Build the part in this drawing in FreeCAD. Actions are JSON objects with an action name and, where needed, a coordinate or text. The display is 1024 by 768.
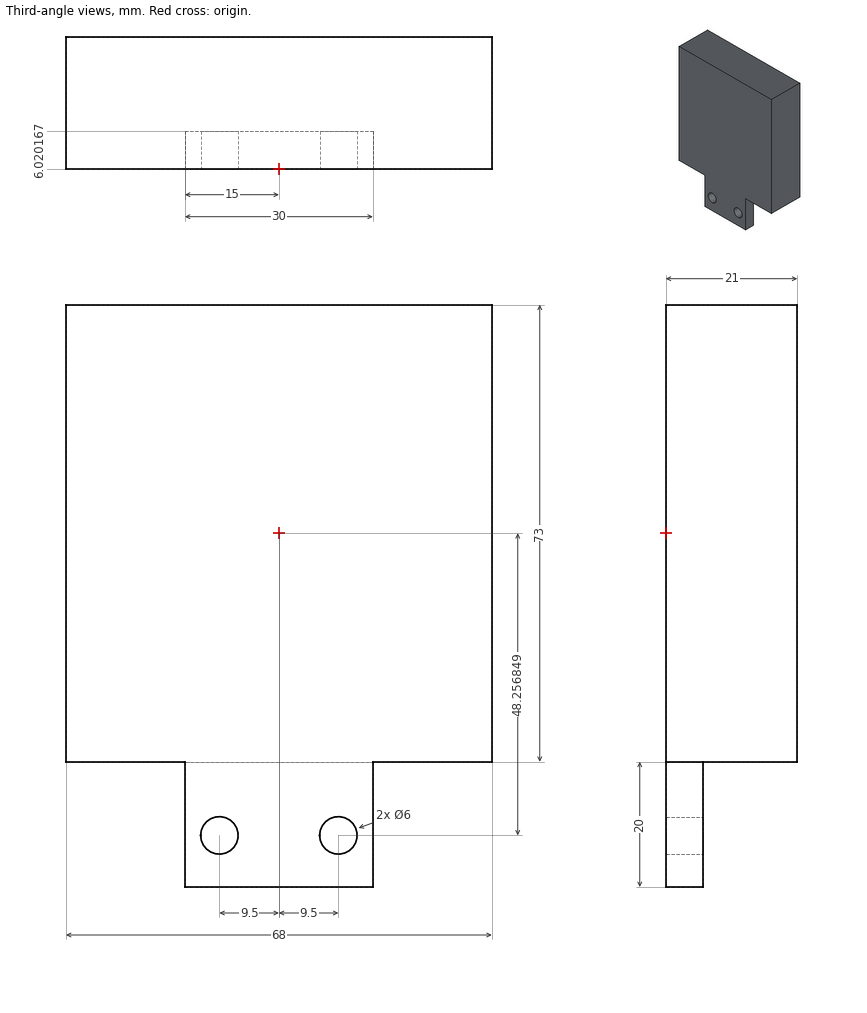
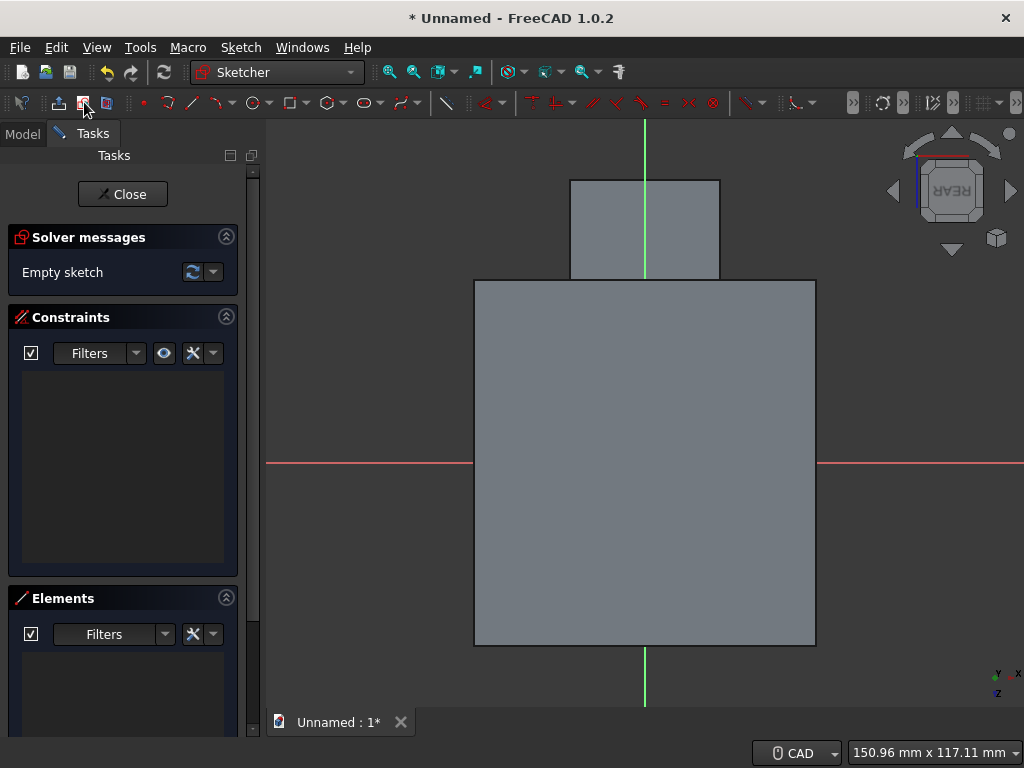
{"action": "key", "text": "q s"}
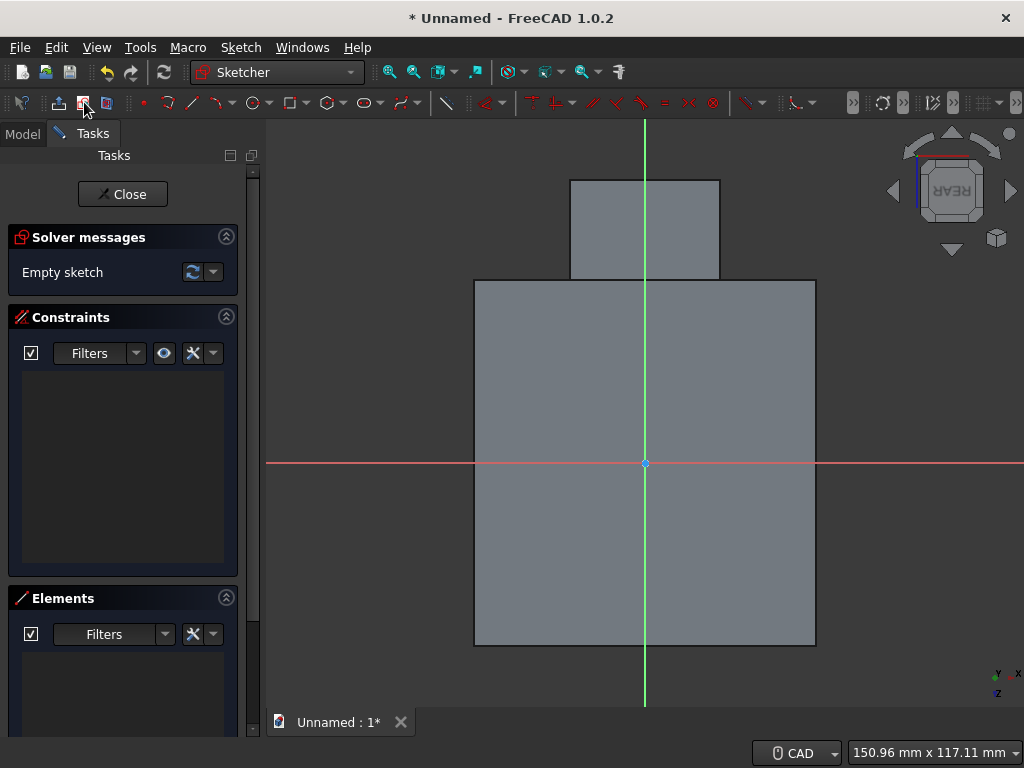
{"action": "scroll", "coordinate": [784, 175], "scroll_direction": "up", "scroll_amount": 2}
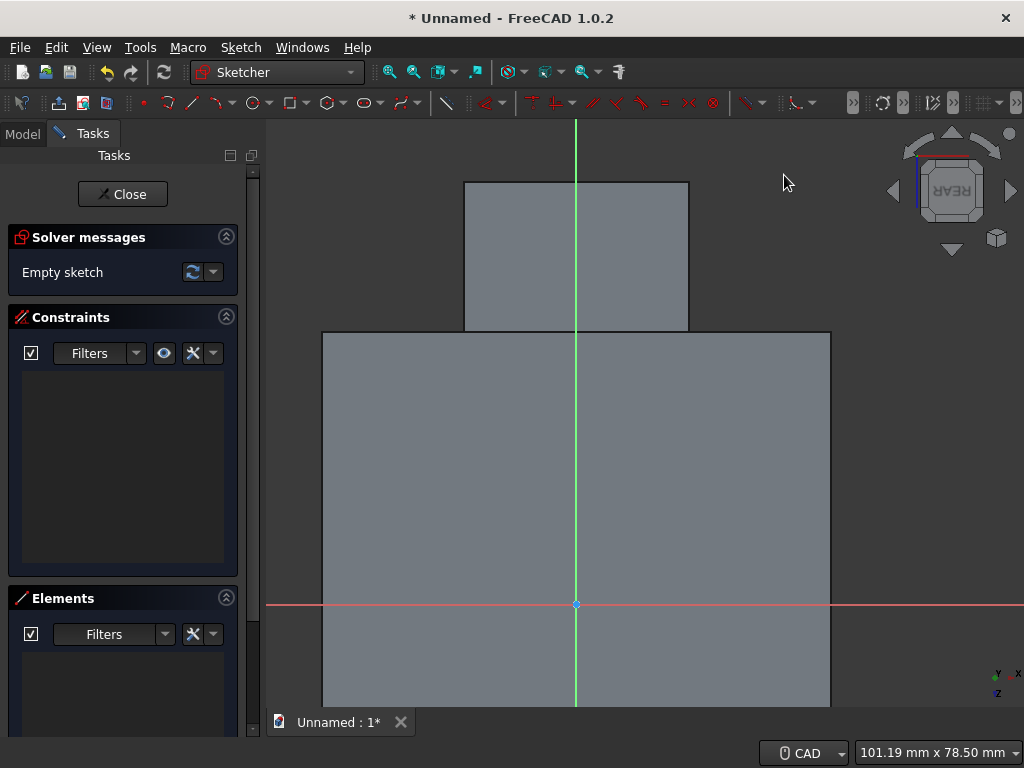
{"action": "key", "text": "g c"}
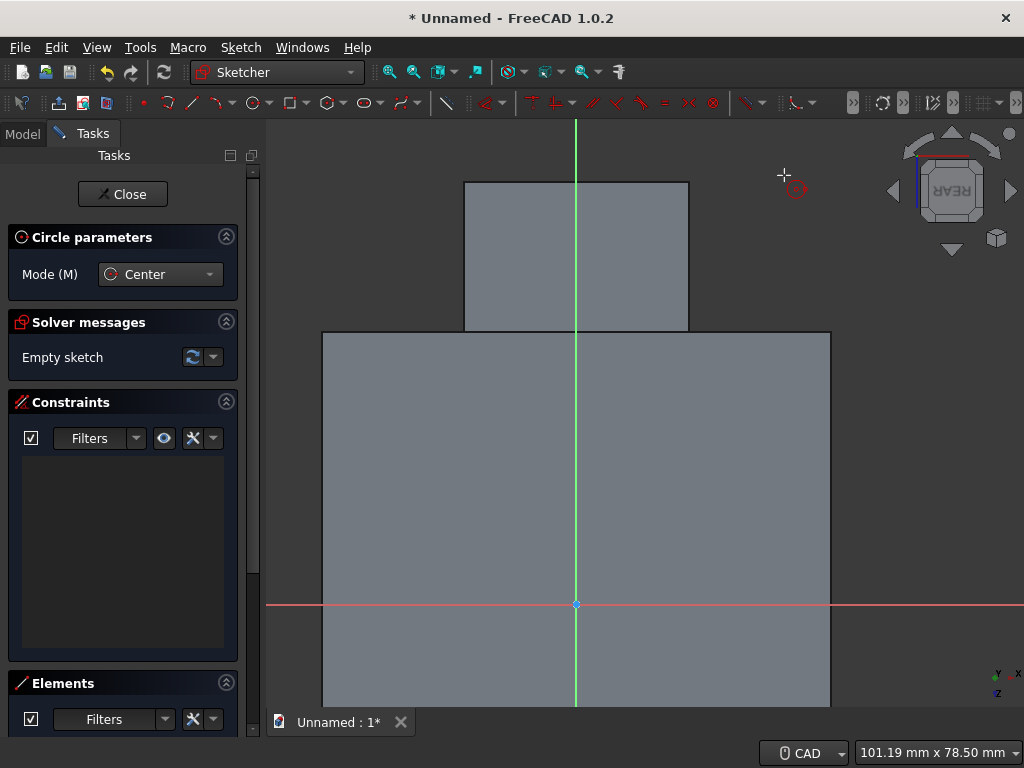
{"action": "left_click", "coordinate": [647, 243]}
{"action": "left_click", "coordinate": [663, 228]}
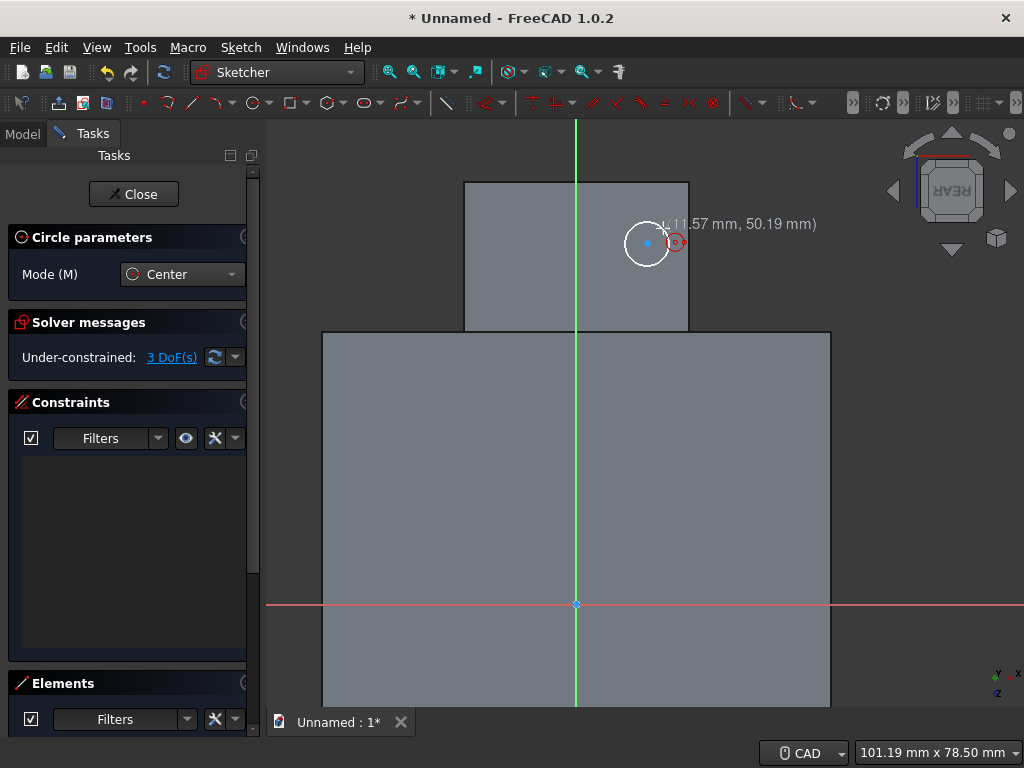
{"action": "left_click", "coordinate": [505, 243]}
{"action": "left_click", "coordinate": [521, 228]}
{"action": "key", "text": "Escape"}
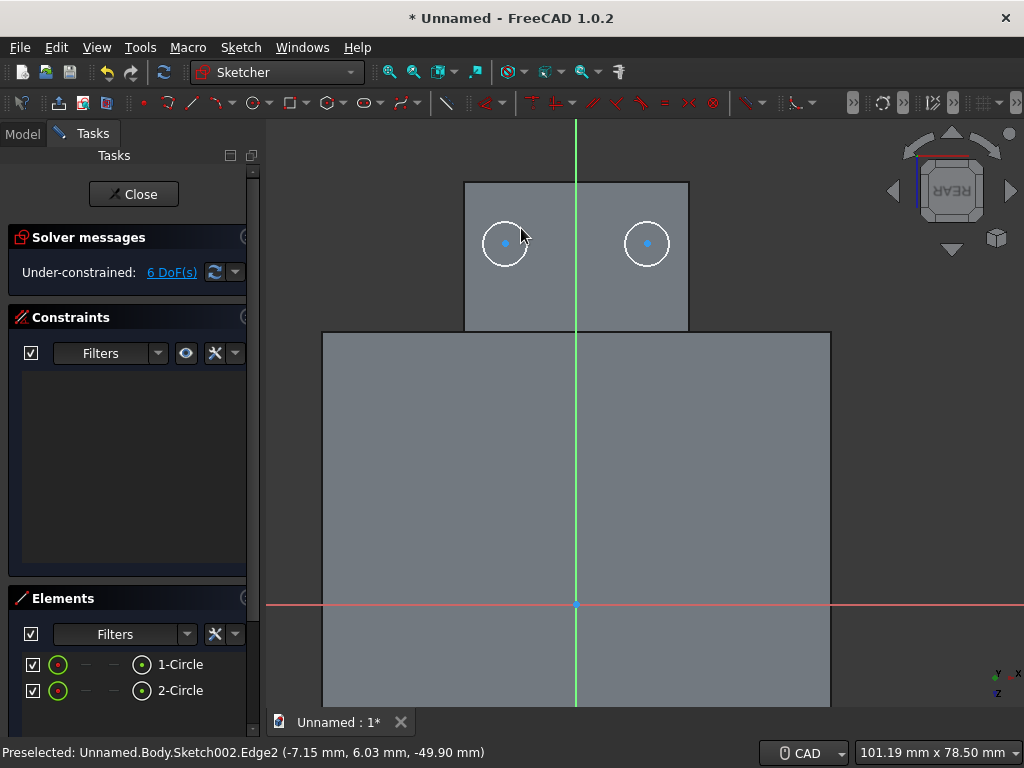
{"action": "left_click", "coordinate": [662, 228]}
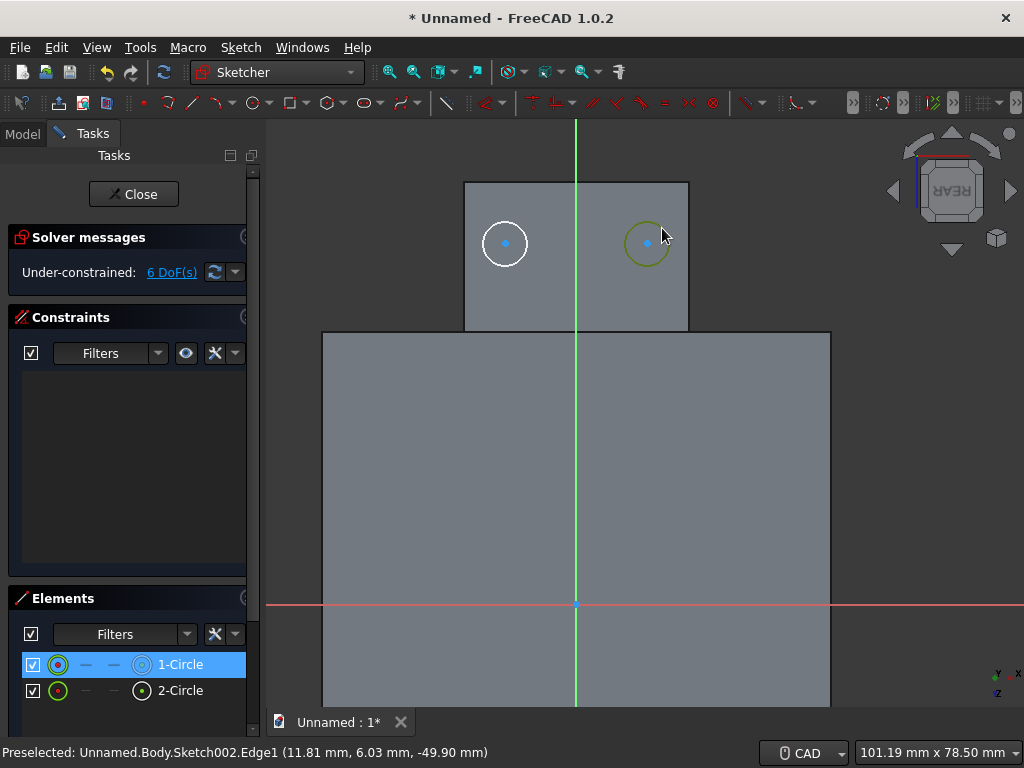
{"action": "left_click", "coordinate": [520, 228]}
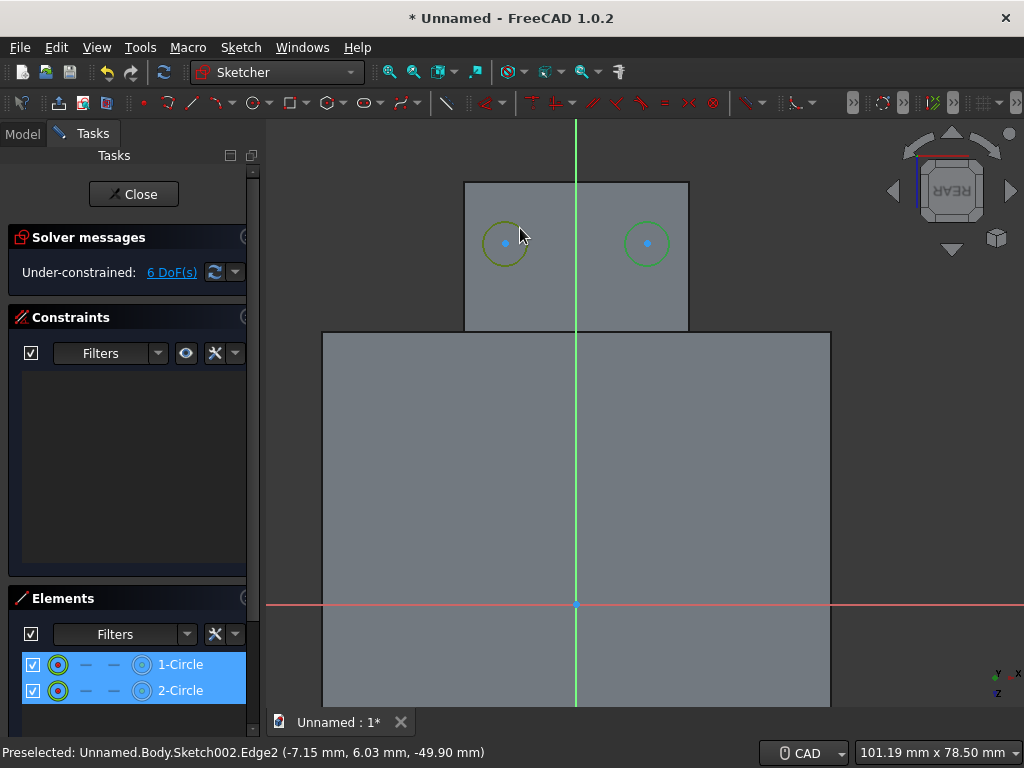
{"action": "key", "text": "e"}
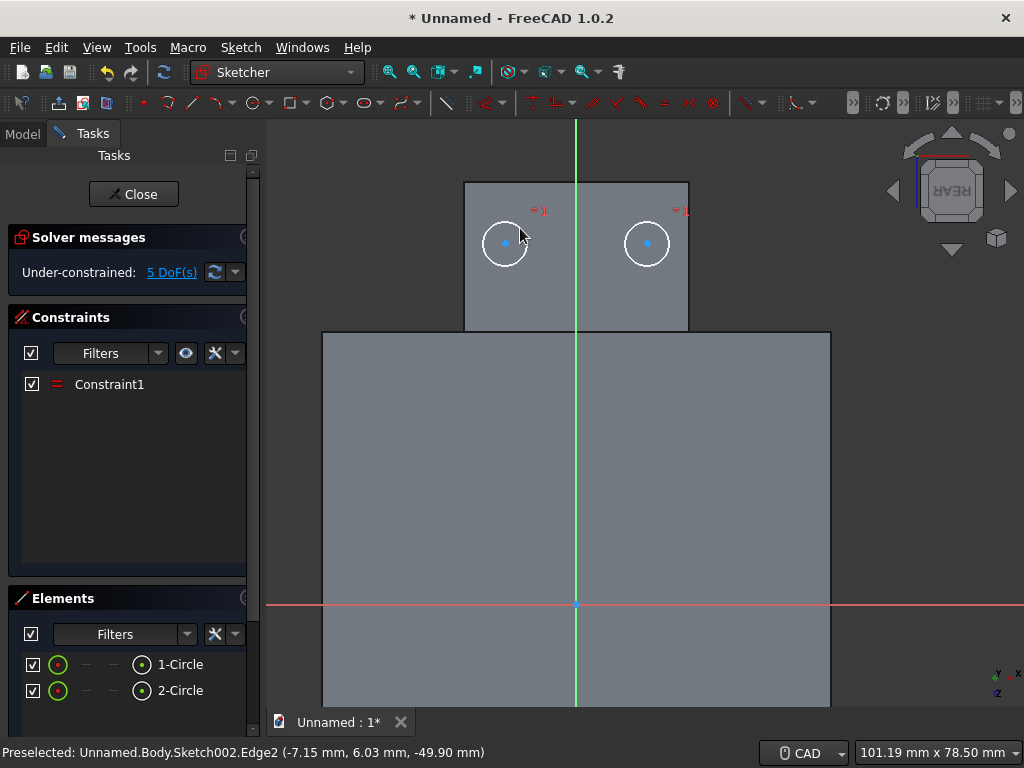
{"action": "left_click", "coordinate": [647, 244]}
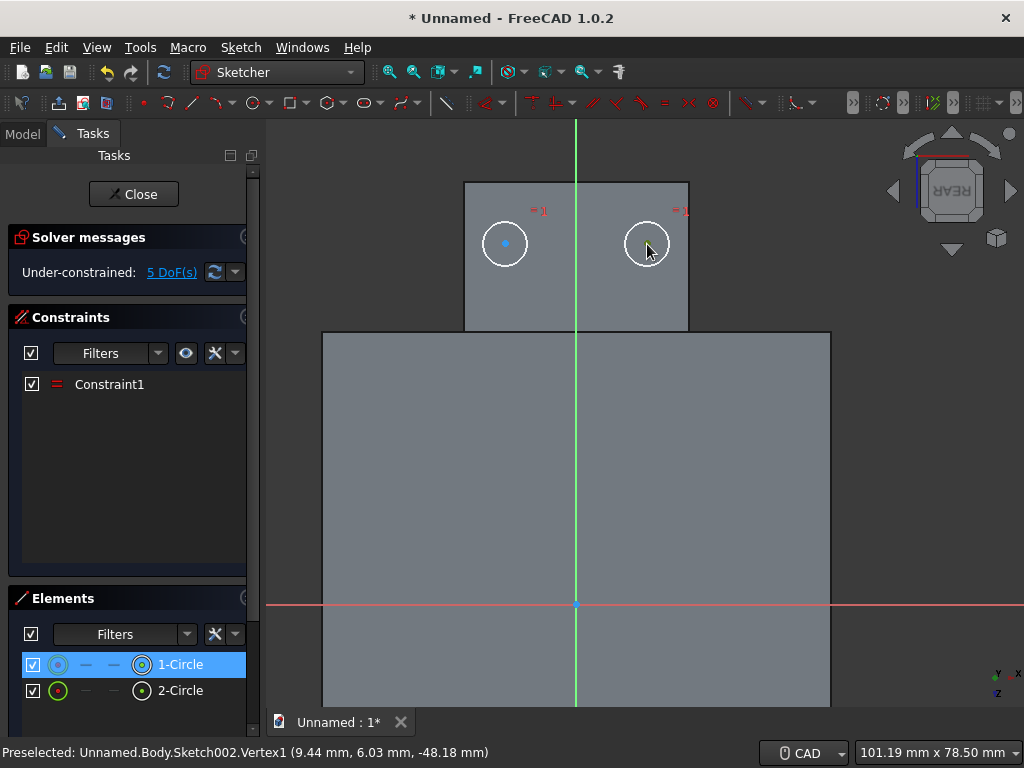
{"action": "left_click", "coordinate": [505, 244]}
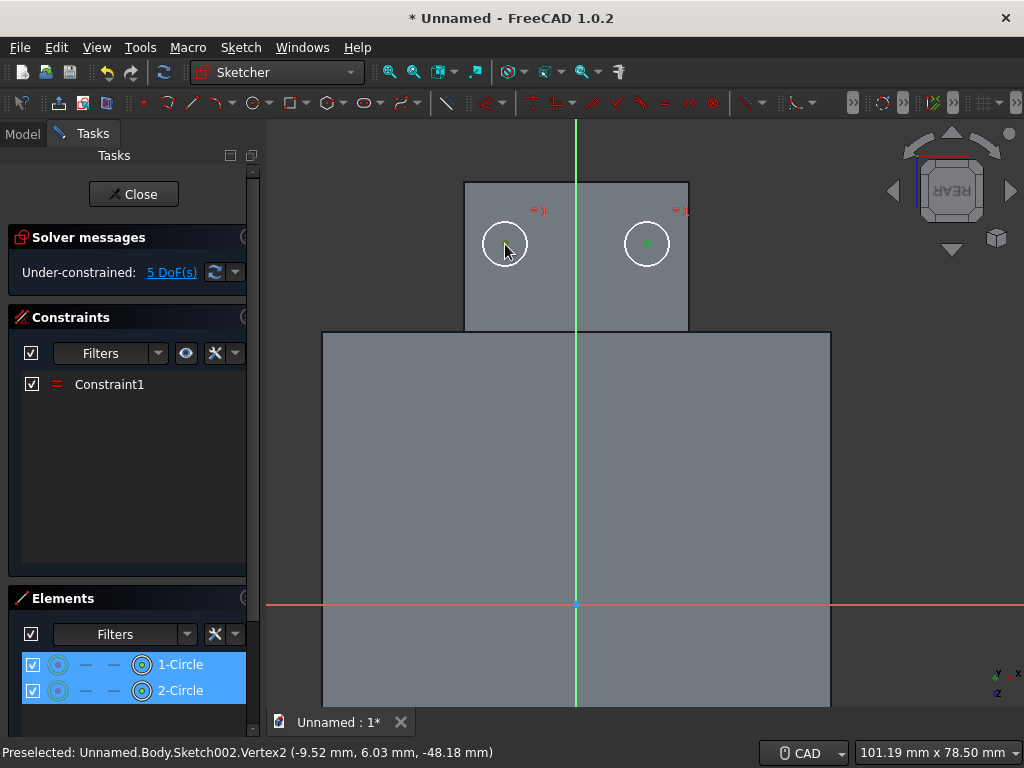
{"action": "key", "text": "h"}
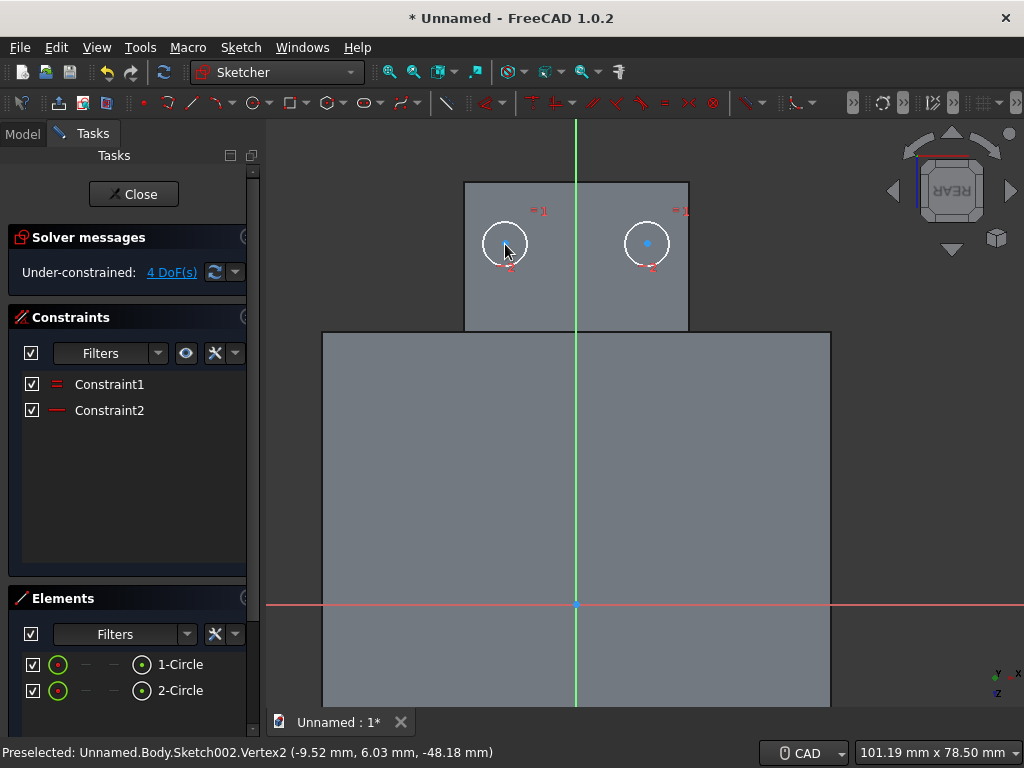
{"action": "key", "text": "d"}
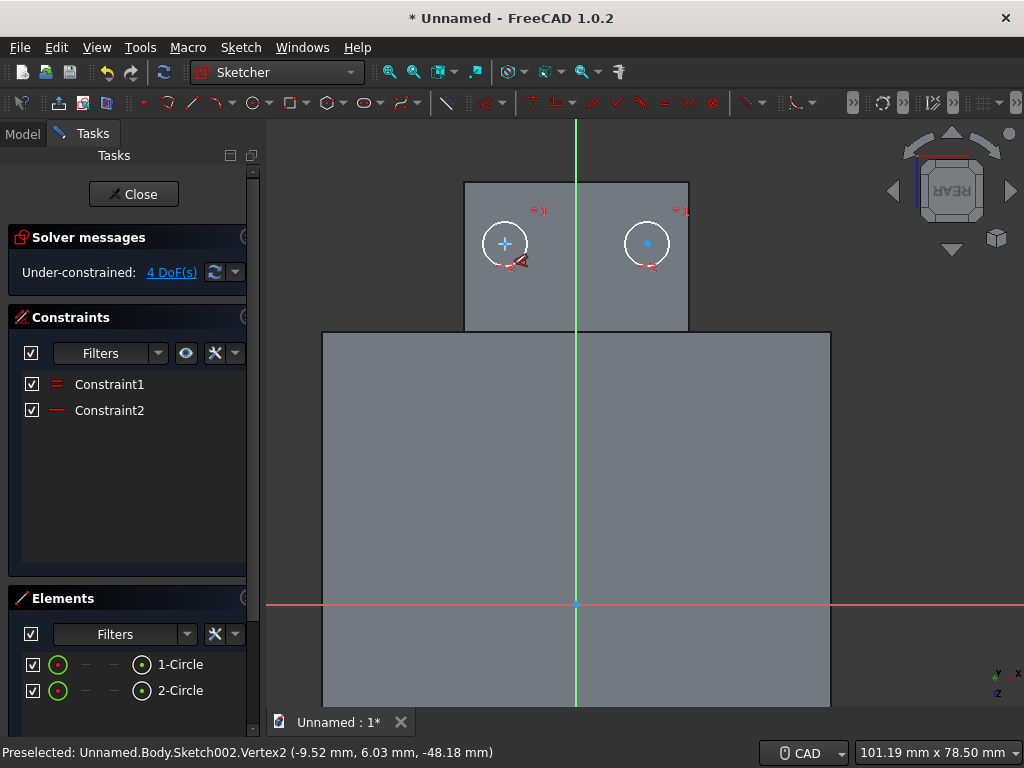
{"action": "left_click", "coordinate": [662, 228]}
{"action": "left_click", "coordinate": [684, 205]}